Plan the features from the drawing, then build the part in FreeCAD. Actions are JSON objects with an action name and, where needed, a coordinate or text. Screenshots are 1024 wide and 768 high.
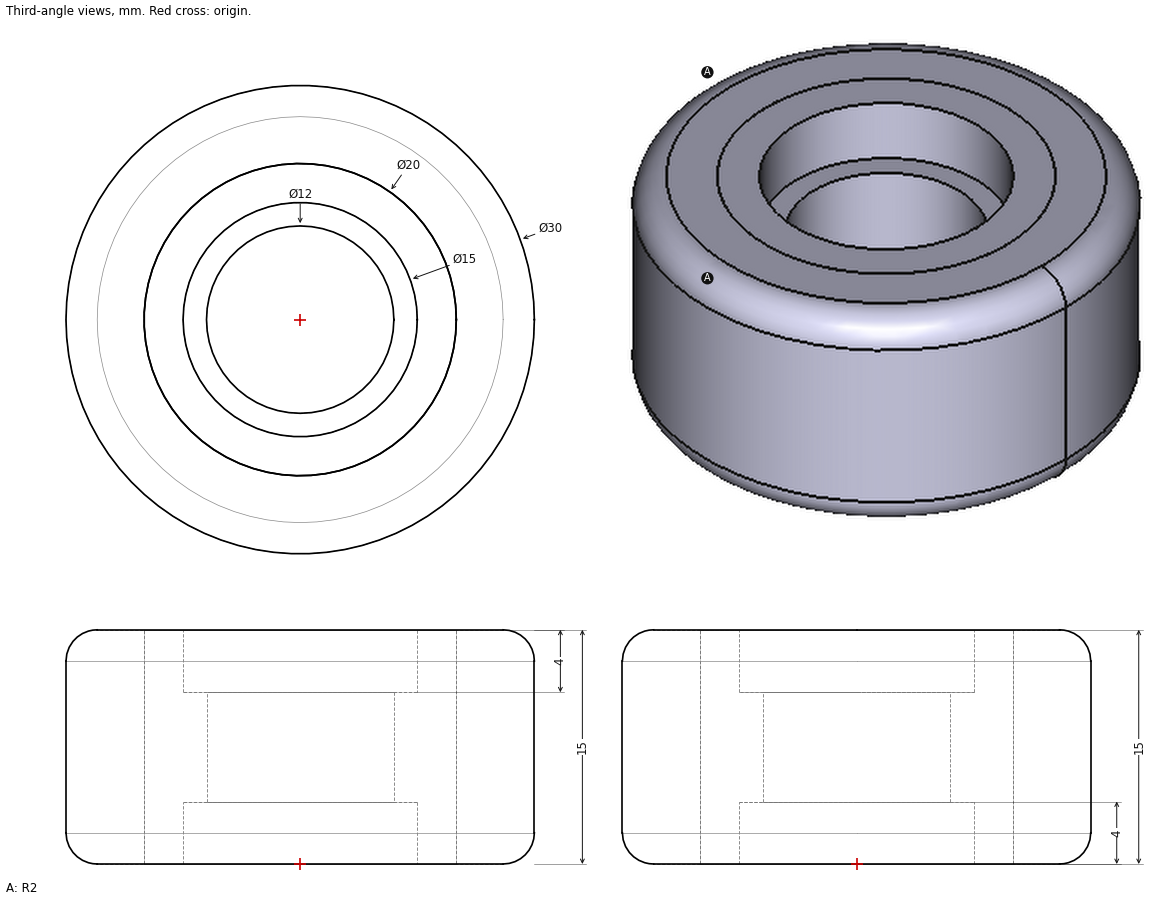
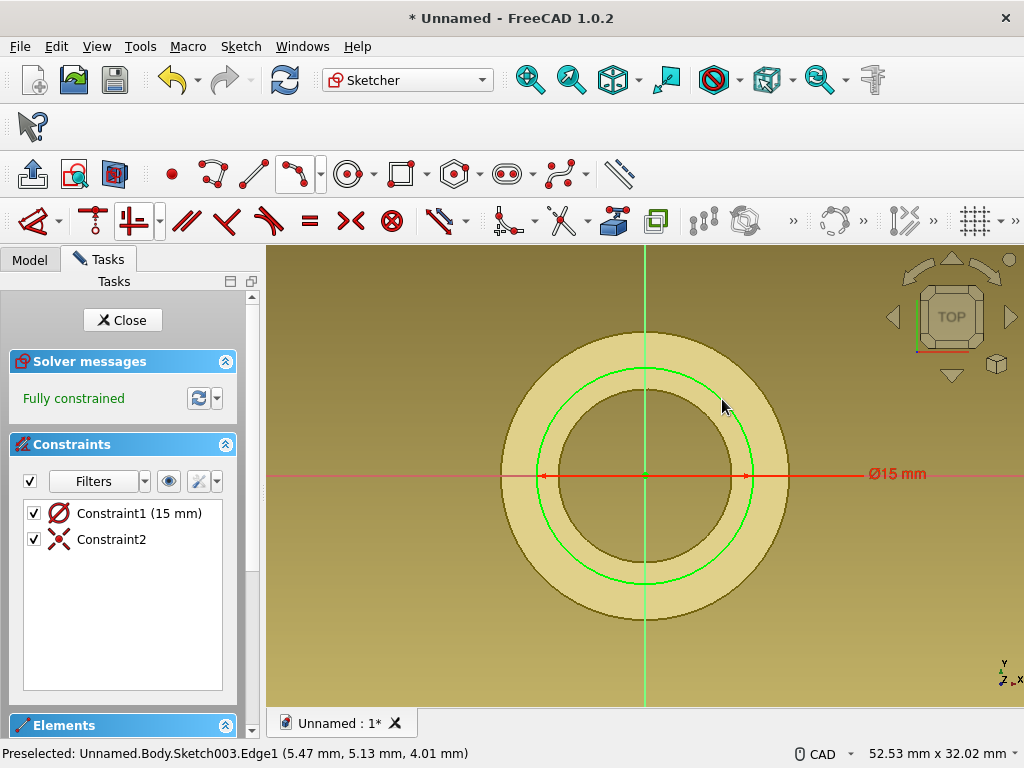
{"action": "left_click", "coordinate": [123, 320]}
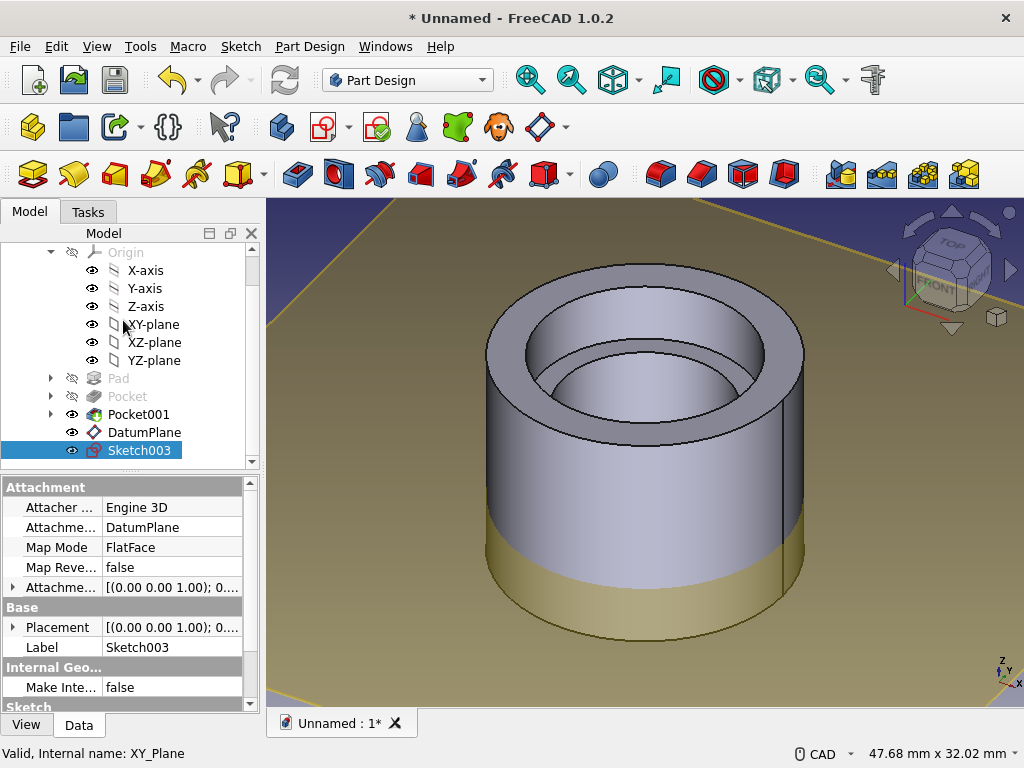
{"action": "left_click", "coordinate": [298, 174]}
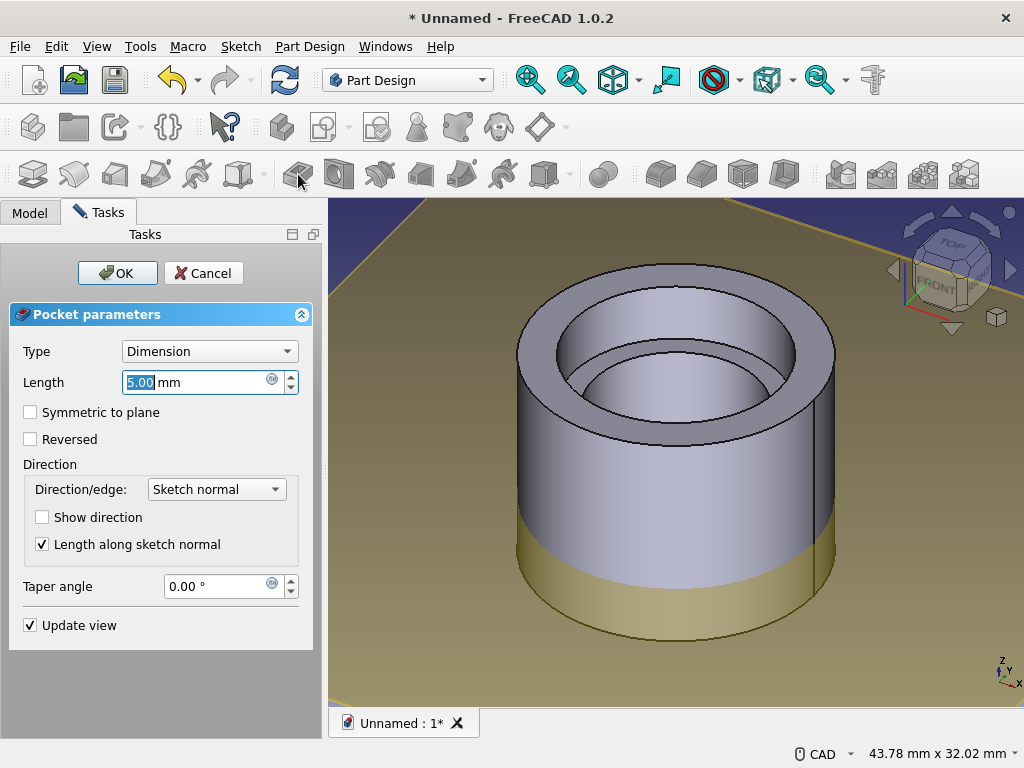
{"action": "type", "text": "4"}
{"action": "key", "text": "Tab"}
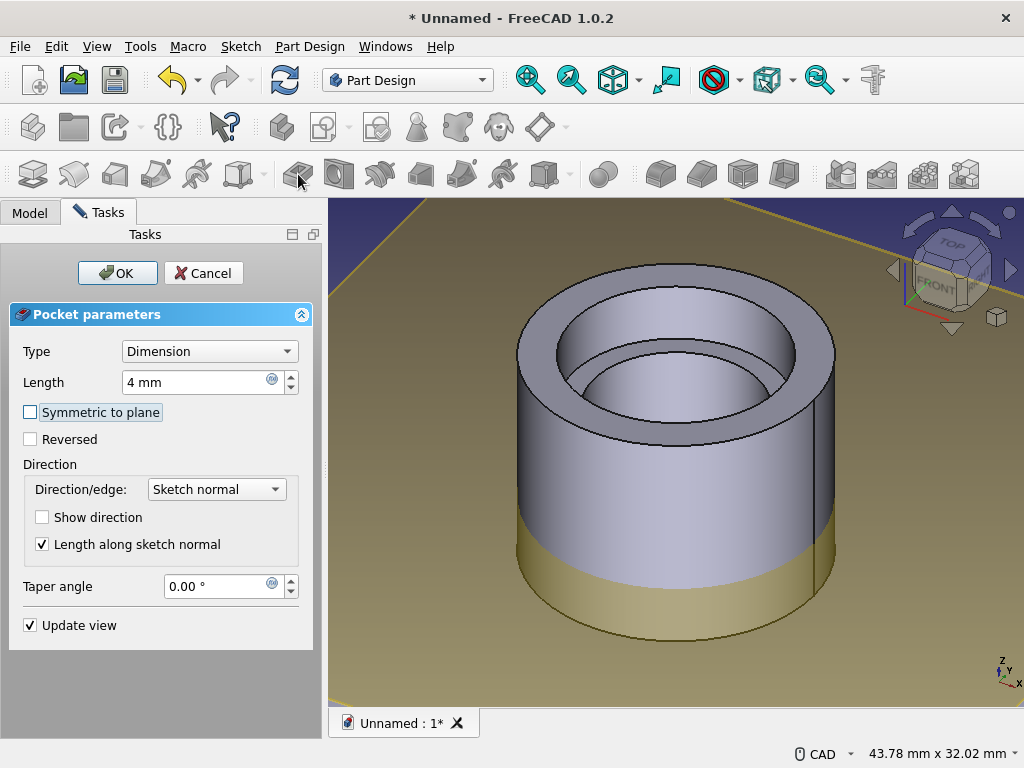
{"action": "left_click", "coordinate": [118, 273]}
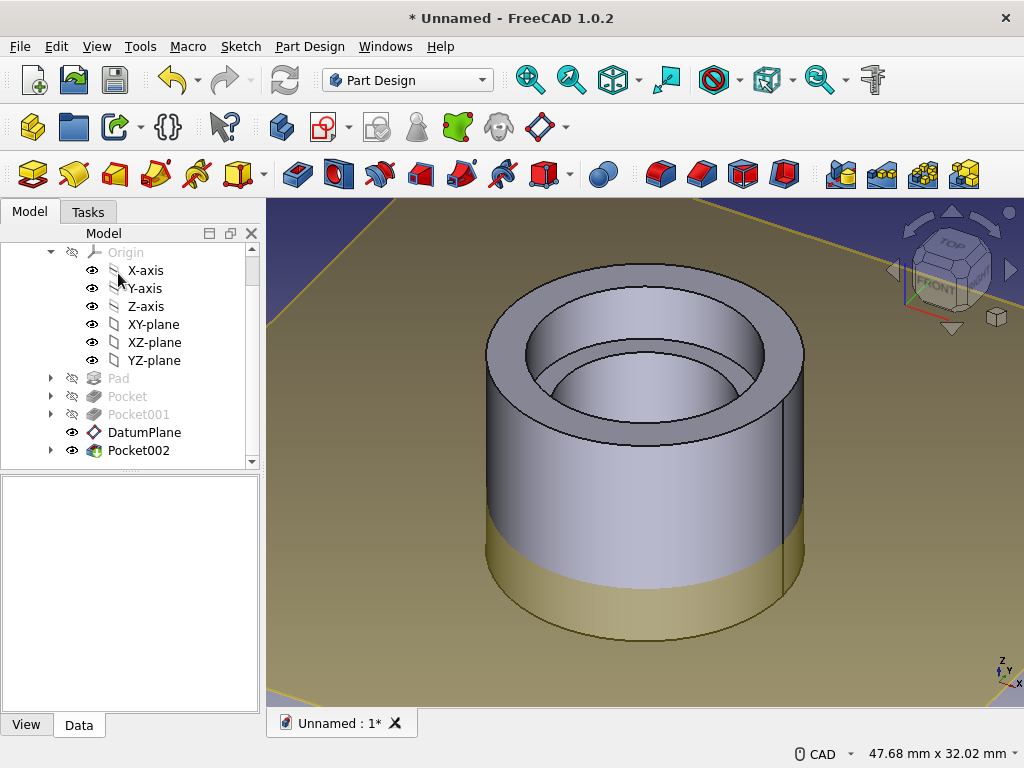
{"action": "left_click", "coordinate": [117, 432]}
{"action": "key", "text": "space"}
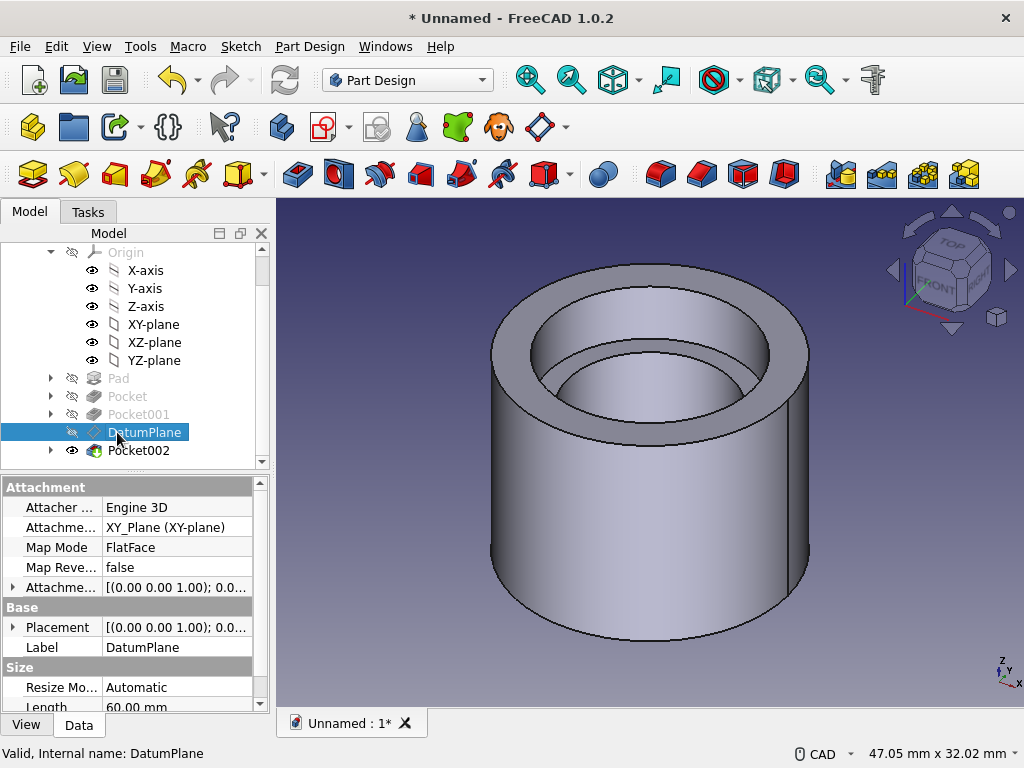
{"action": "left_click", "coordinate": [316, 667]}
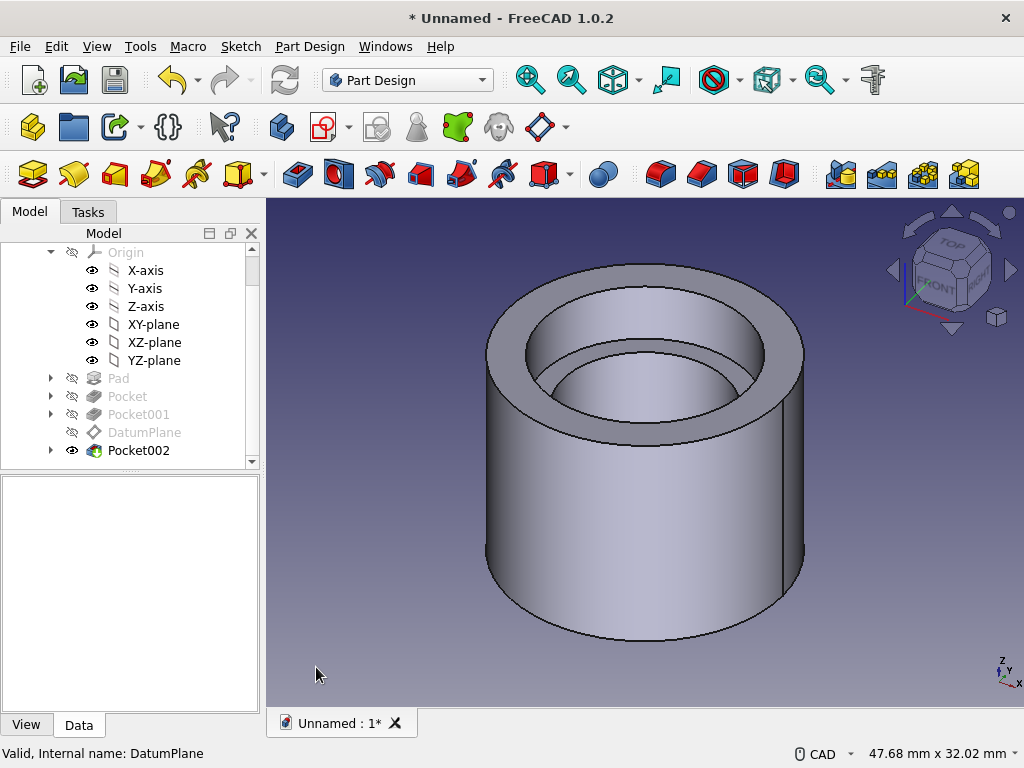
{"action": "left_click", "coordinate": [282, 128]}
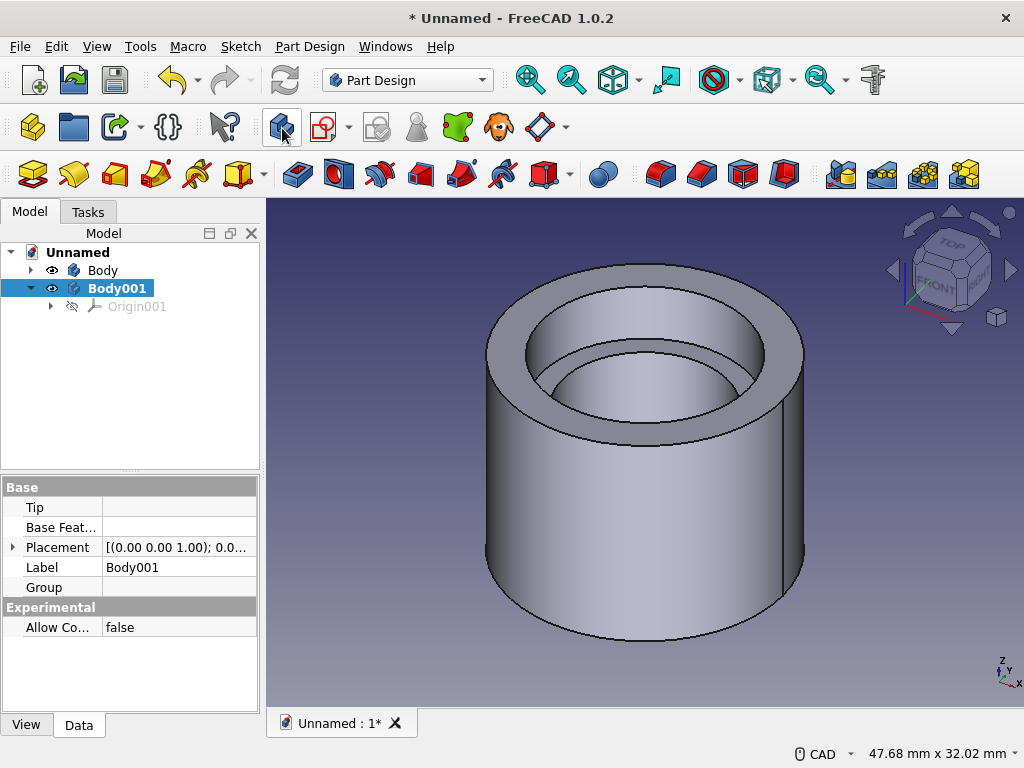
{"action": "left_click", "coordinate": [51, 306]}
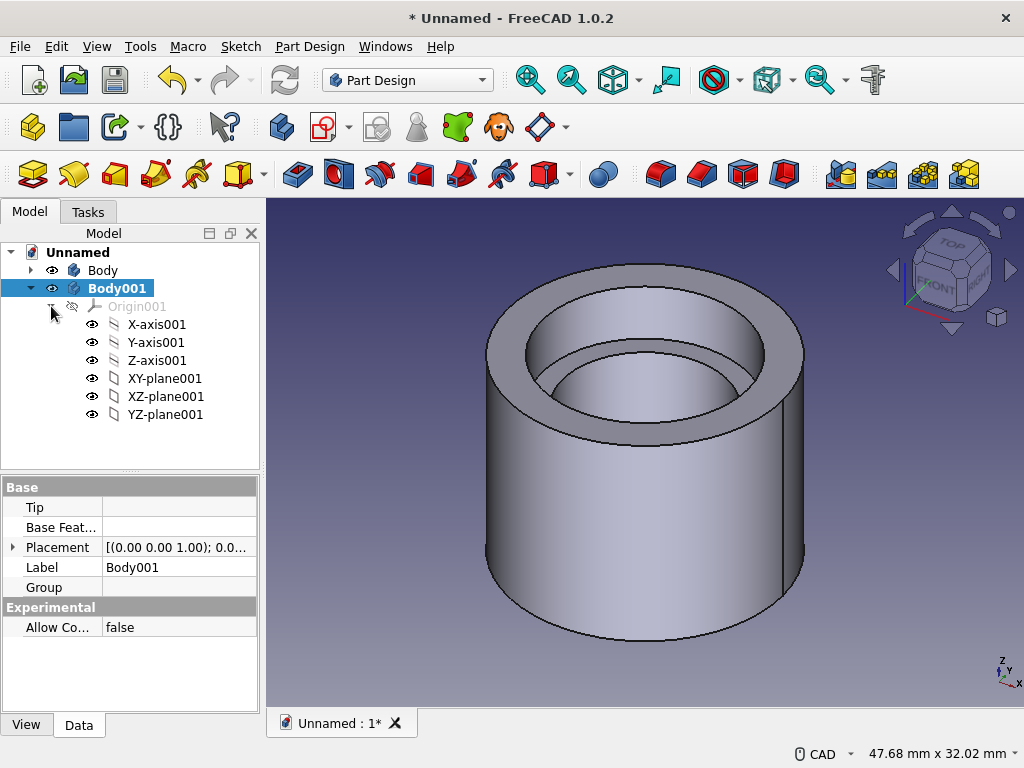
{"action": "left_click", "coordinate": [137, 378]}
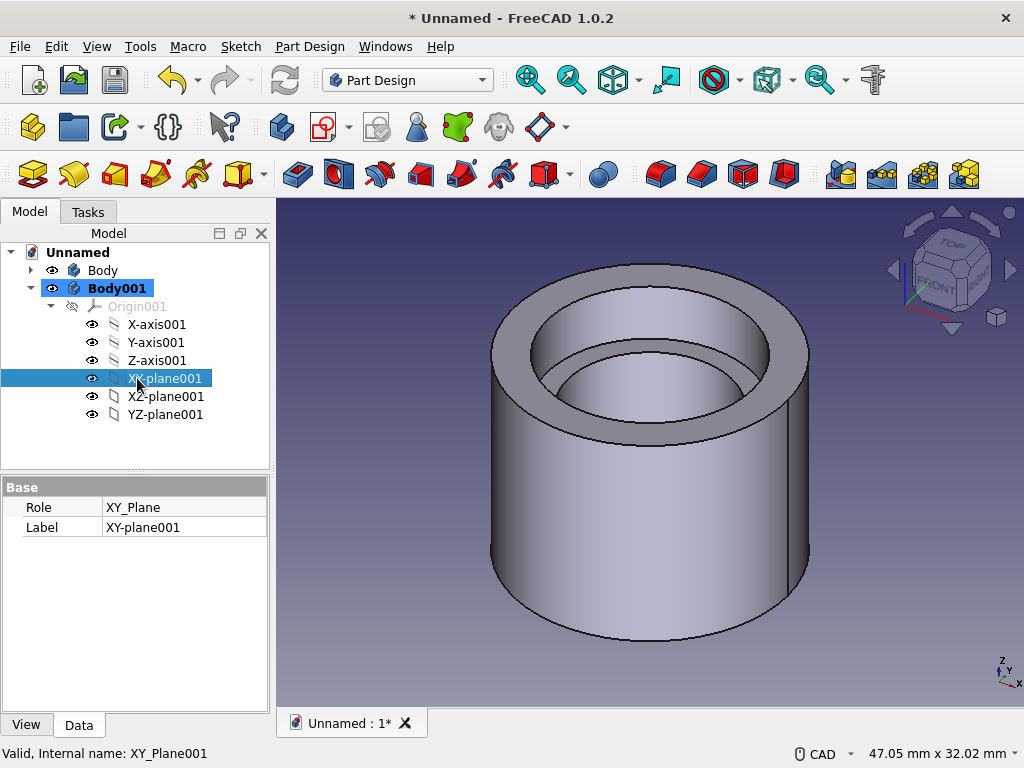
{"action": "left_click", "coordinate": [540, 128]}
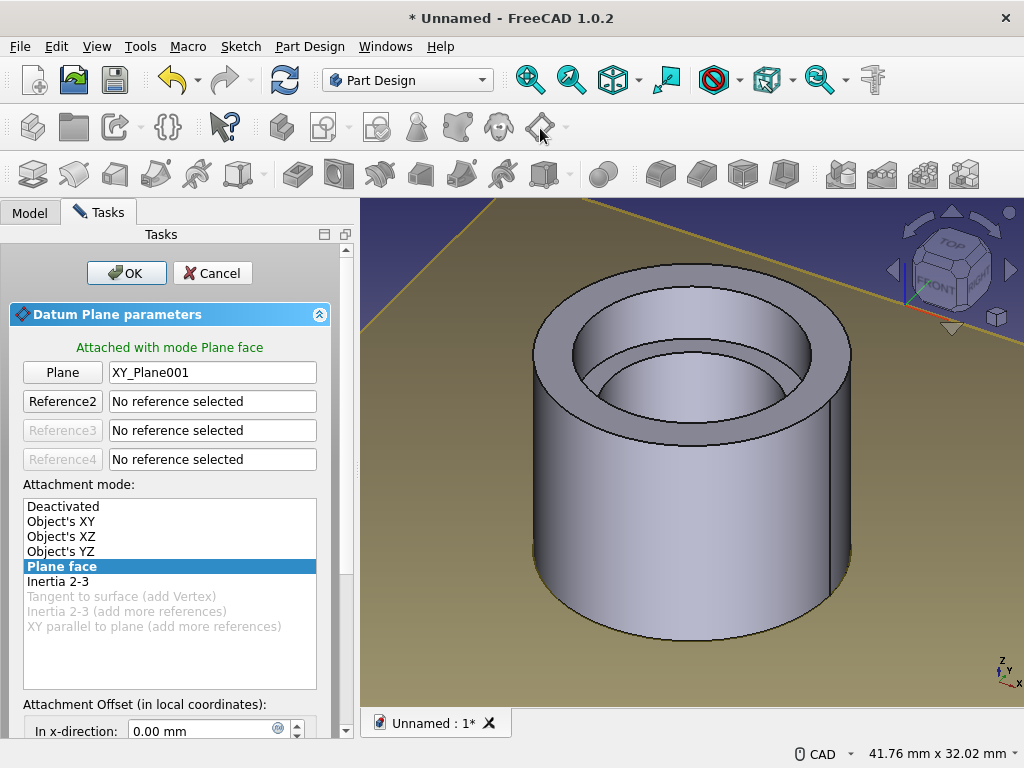
{"action": "scroll", "coordinate": [346, 491], "scroll_direction": "down", "scroll_amount": 3}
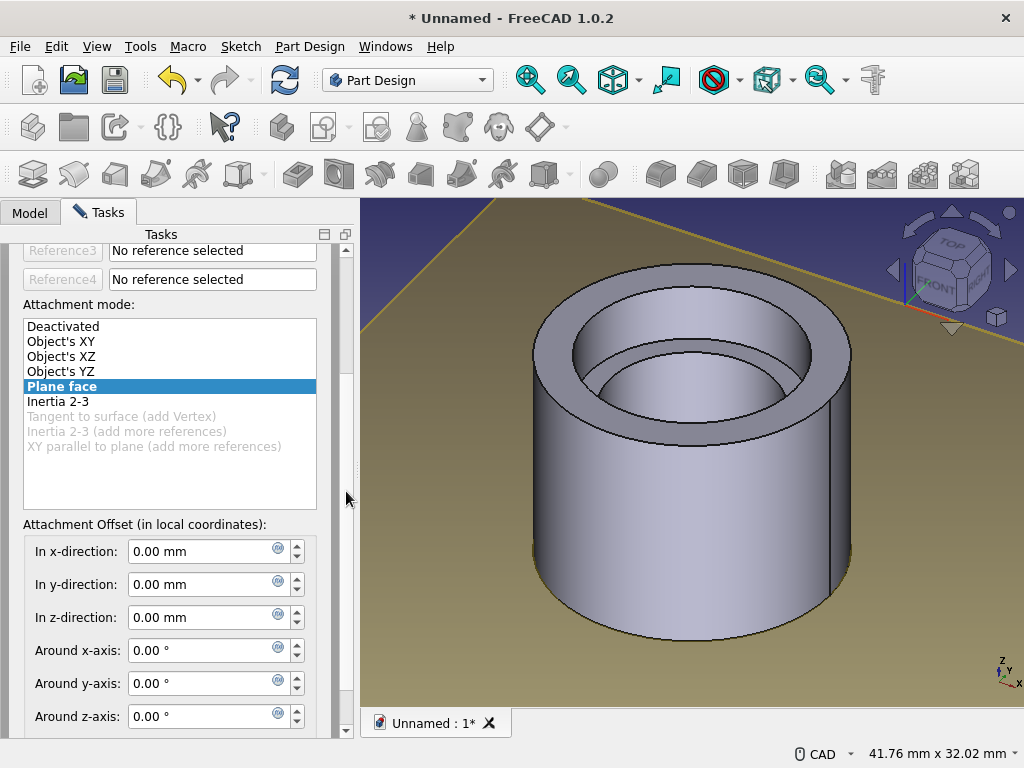
{"action": "triple_click", "coordinate": [210, 618]}